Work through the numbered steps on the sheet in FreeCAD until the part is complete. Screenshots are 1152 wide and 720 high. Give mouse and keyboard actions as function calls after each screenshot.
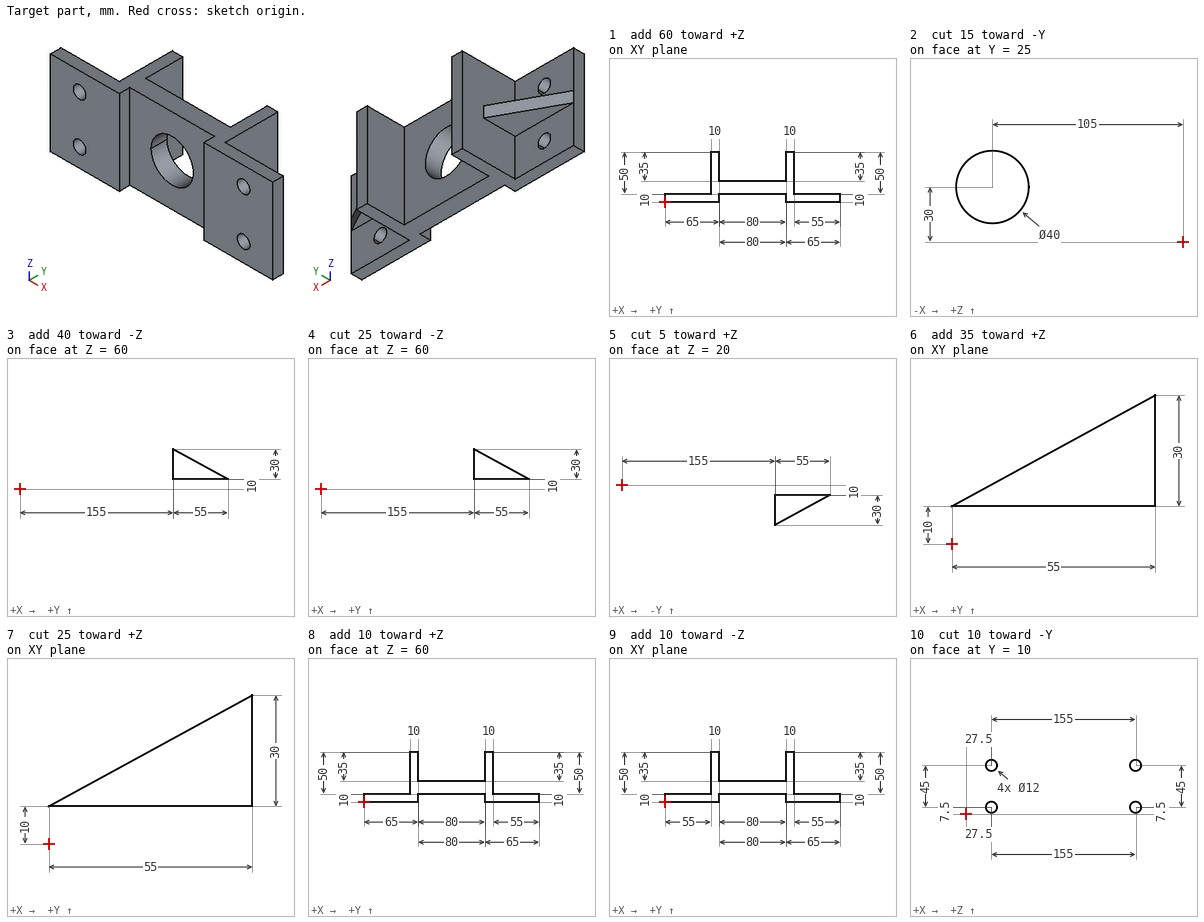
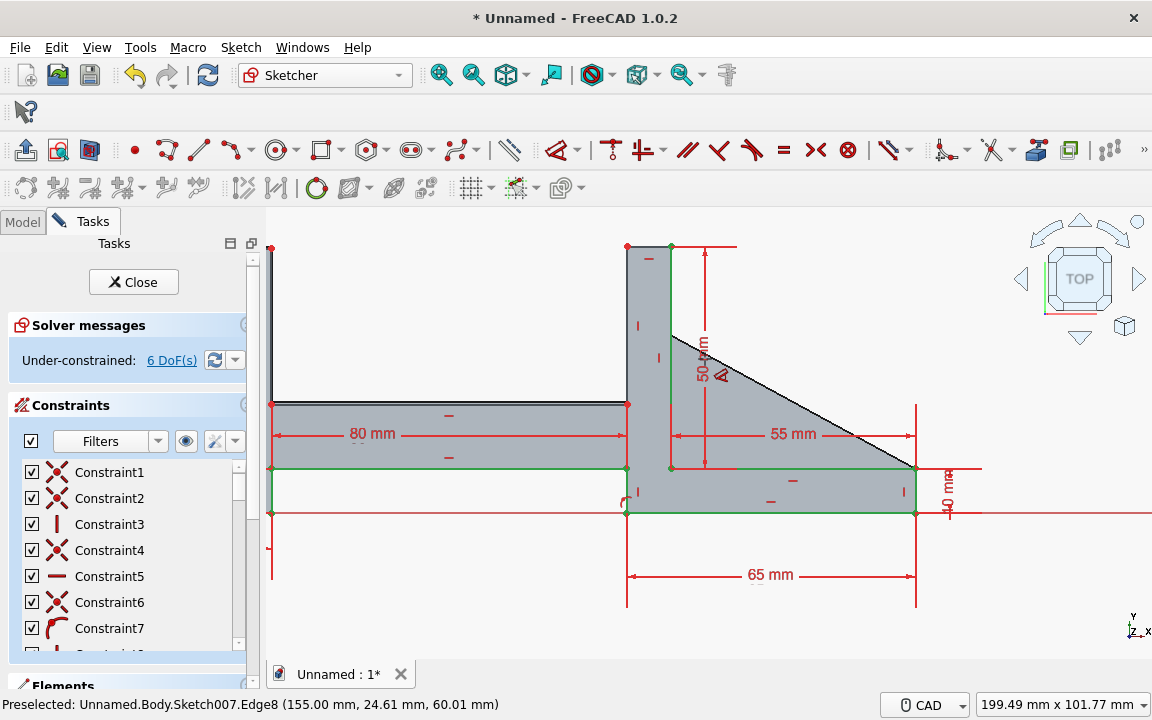
click(658, 247)
click(649, 281)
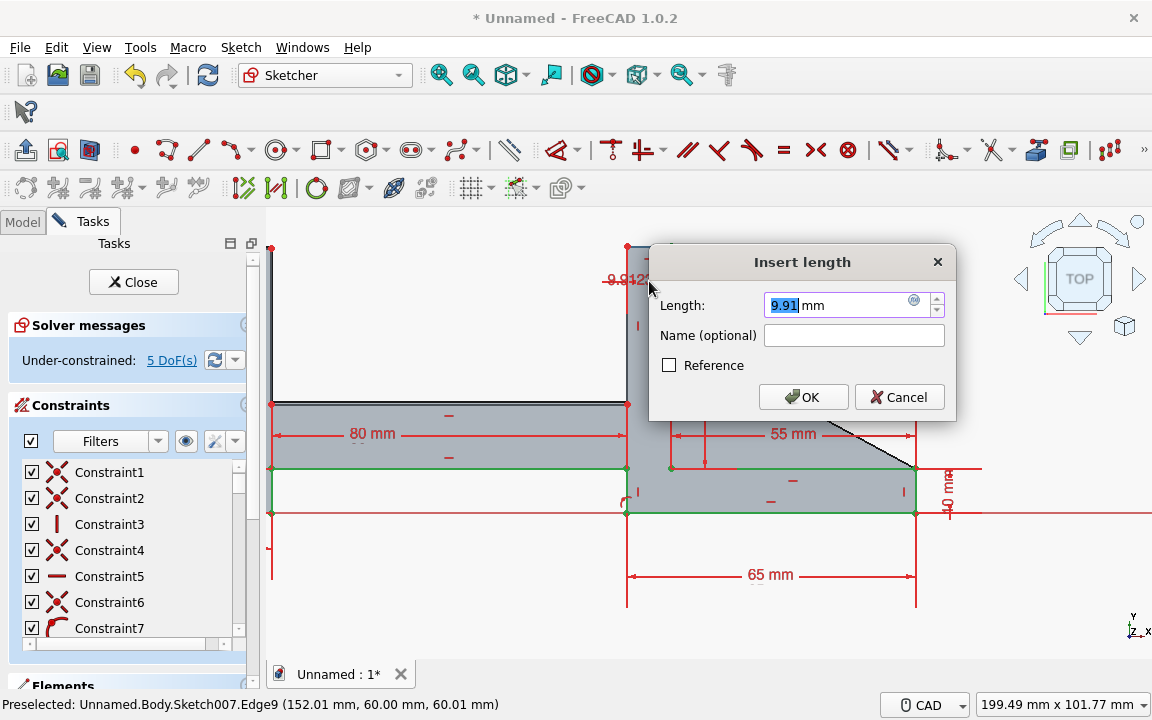
text(10)
key(Return)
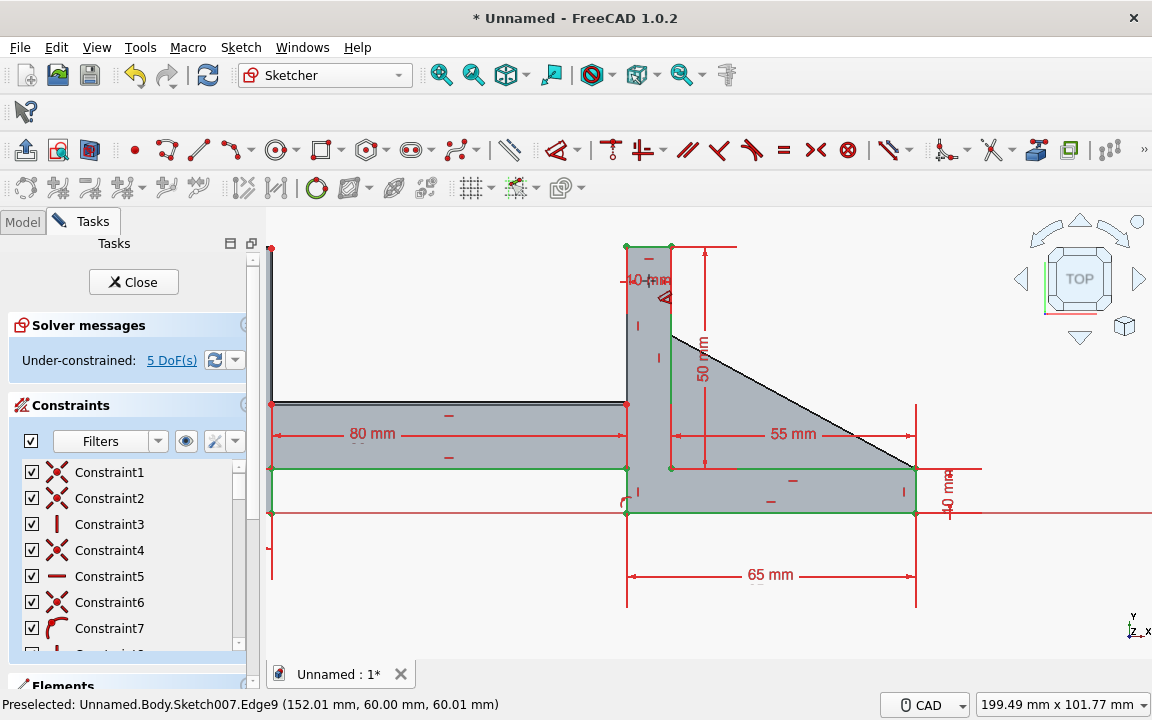
click(627, 294)
click(593, 326)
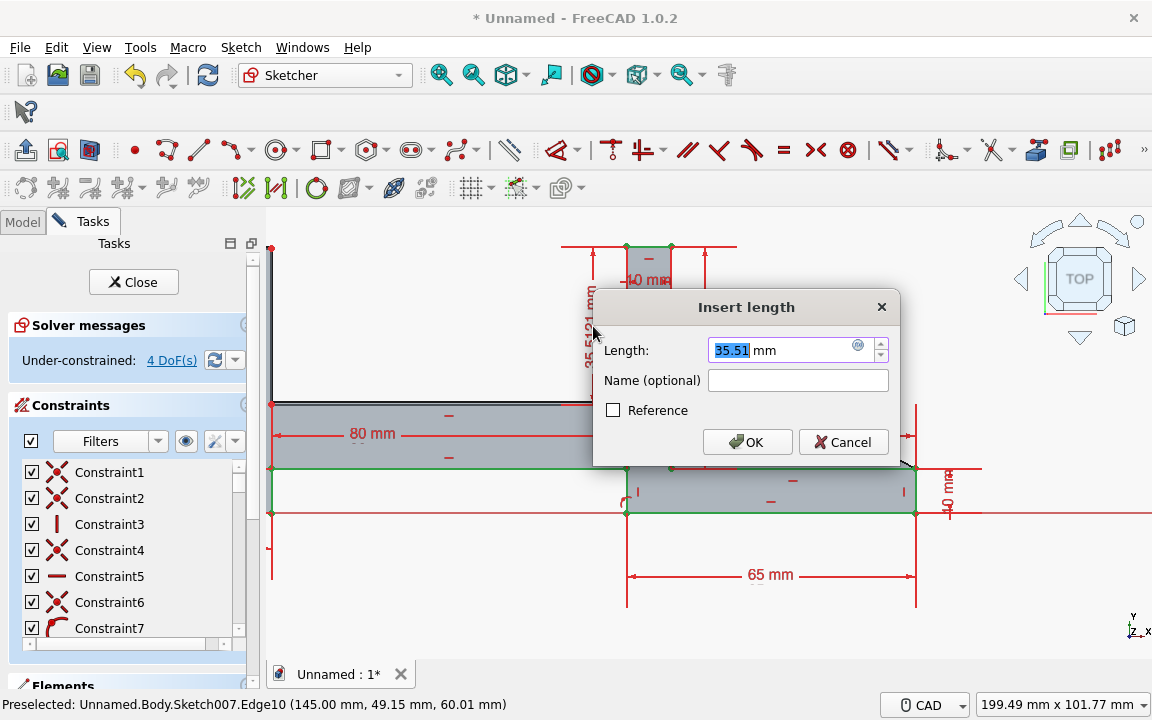
text(35)
key(Return)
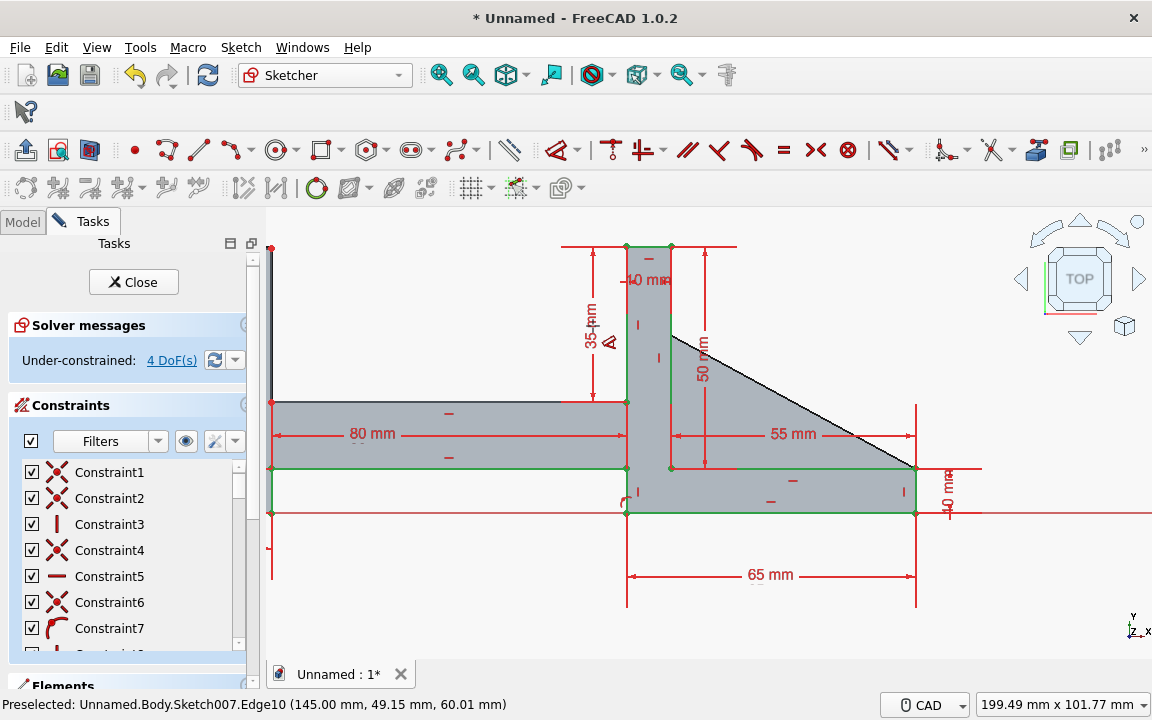
click(520, 402)
click(460, 436)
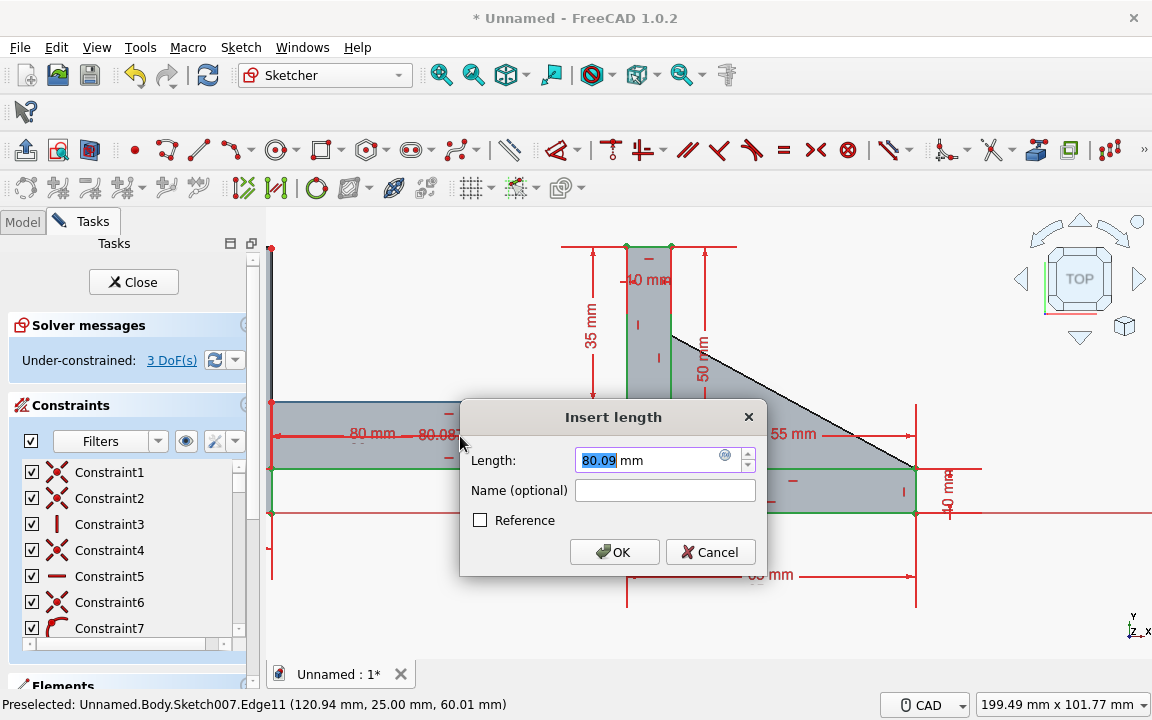
text(80)
key(Return)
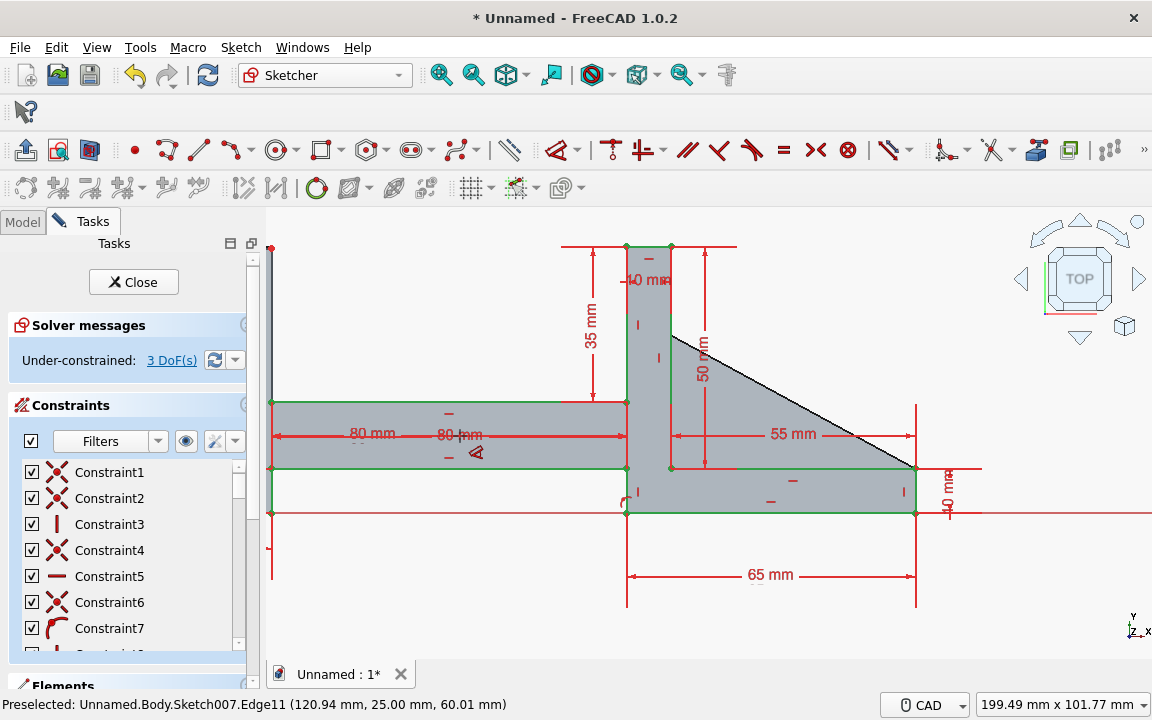
scroll(873, 497, down, 3)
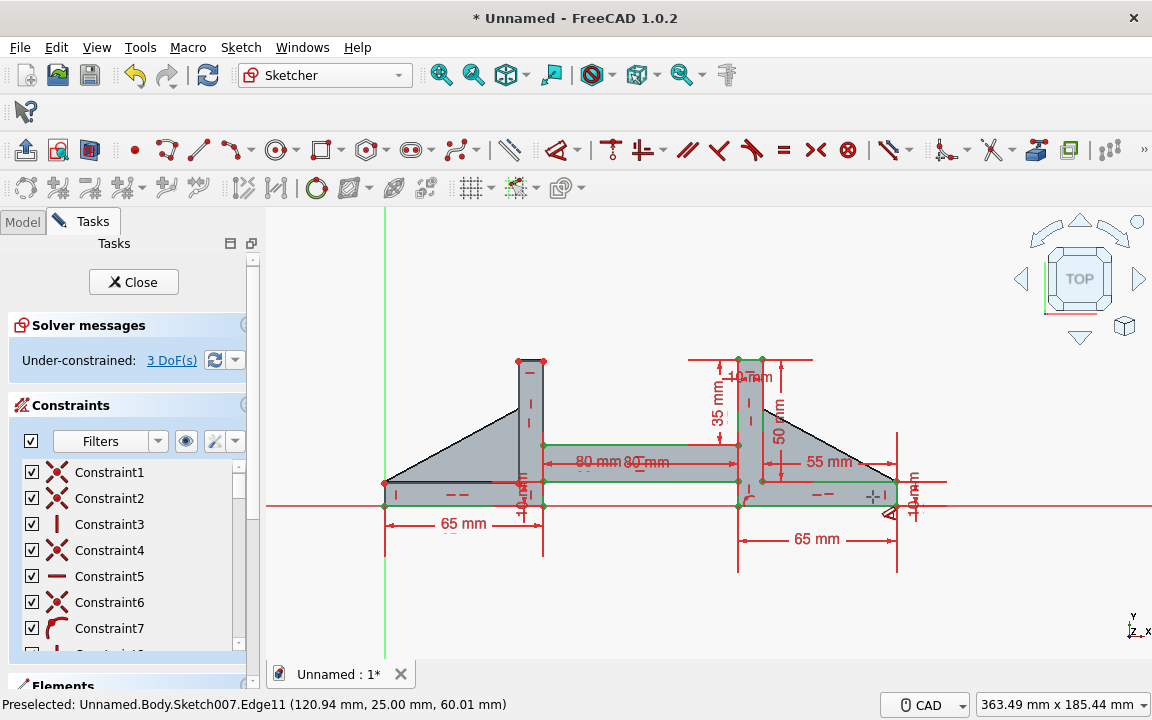
click(543, 420)
click(577, 403)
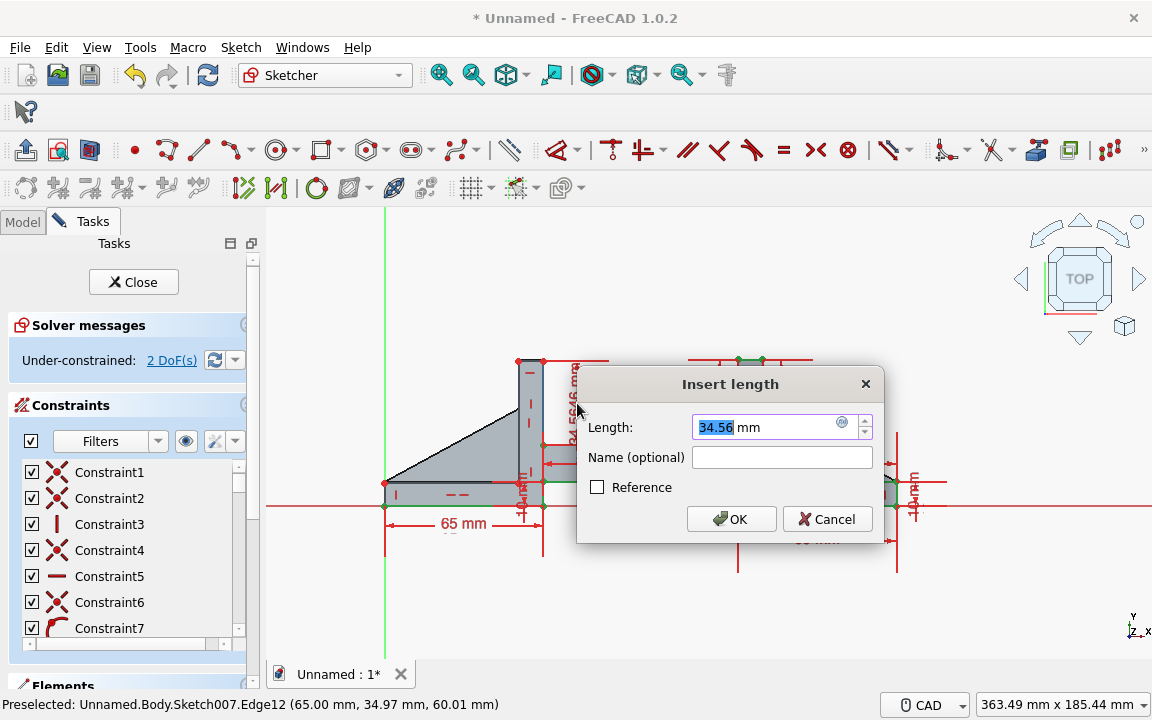
text(35)
key(Return)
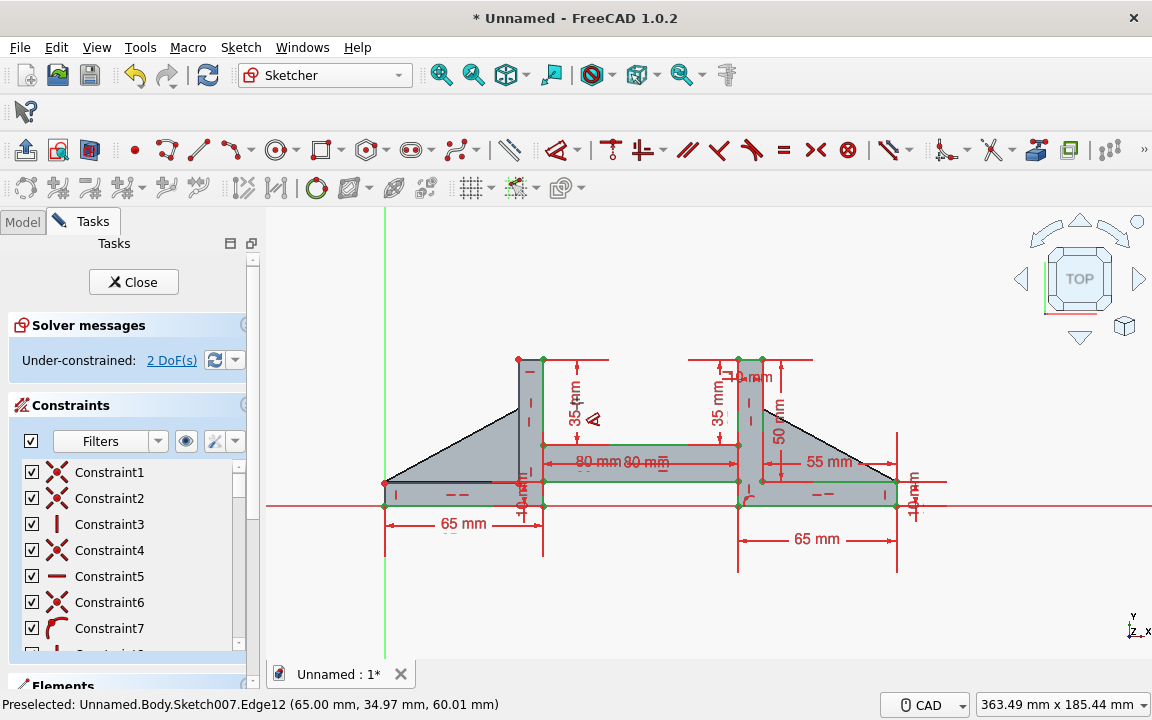
scroll(533, 360, up, 3)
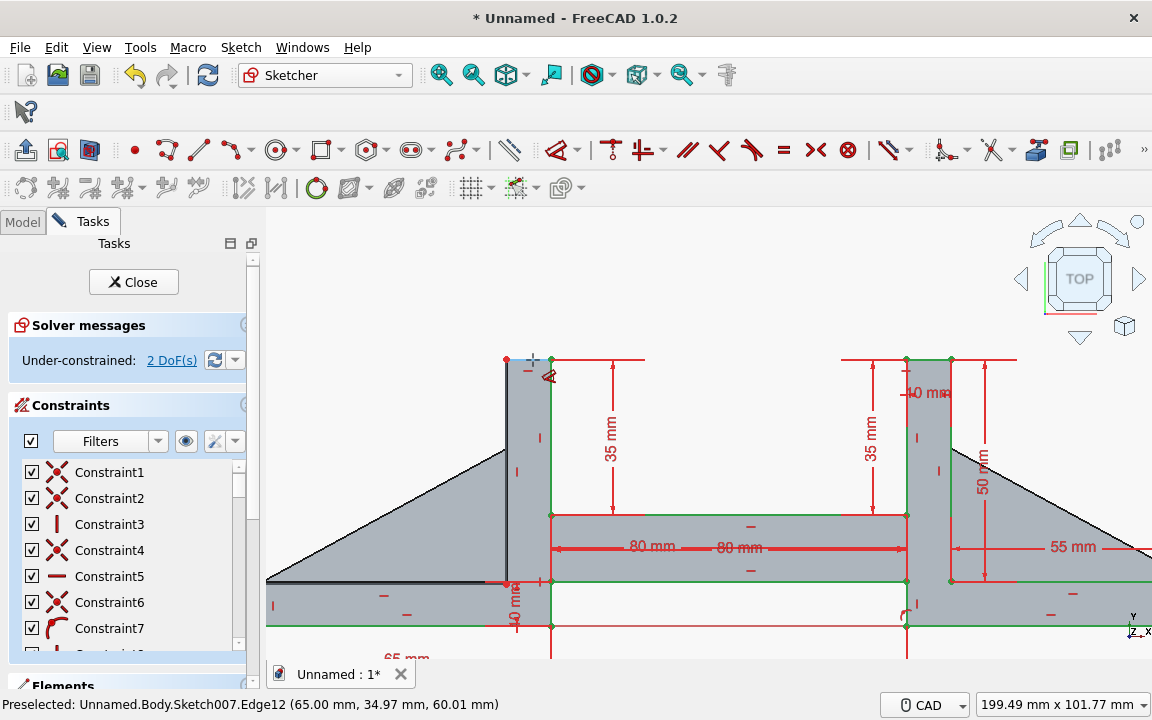
click(533, 360)
click(529, 326)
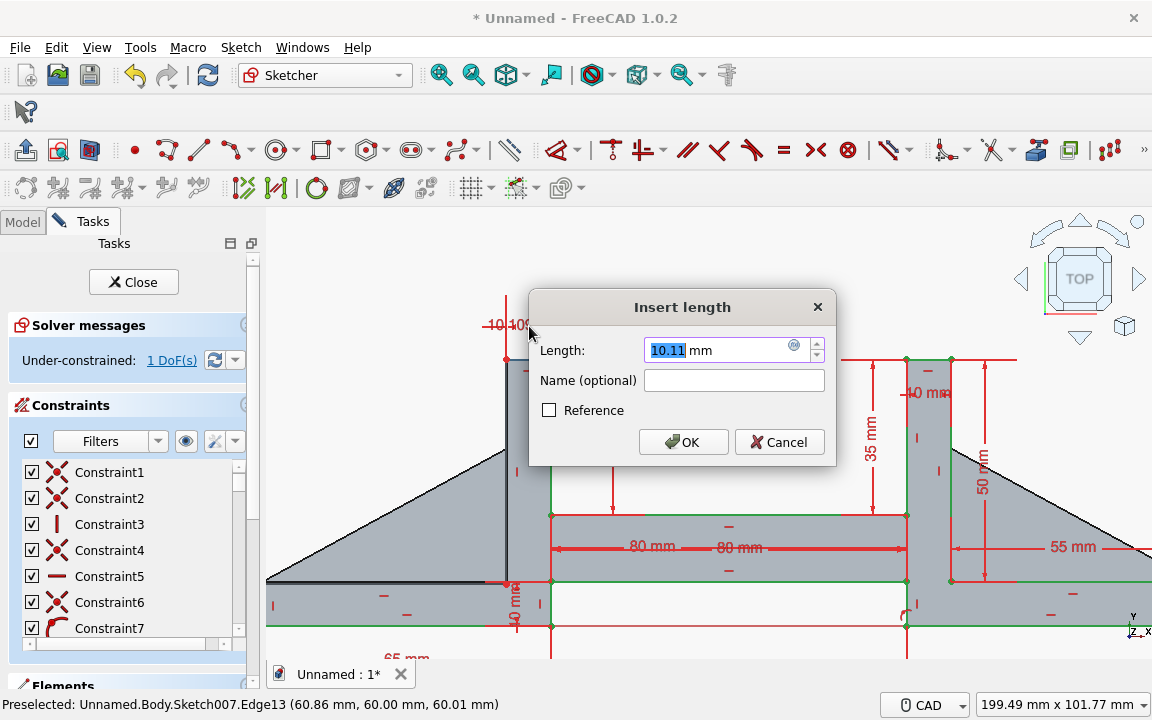
text(10)
key(Return)